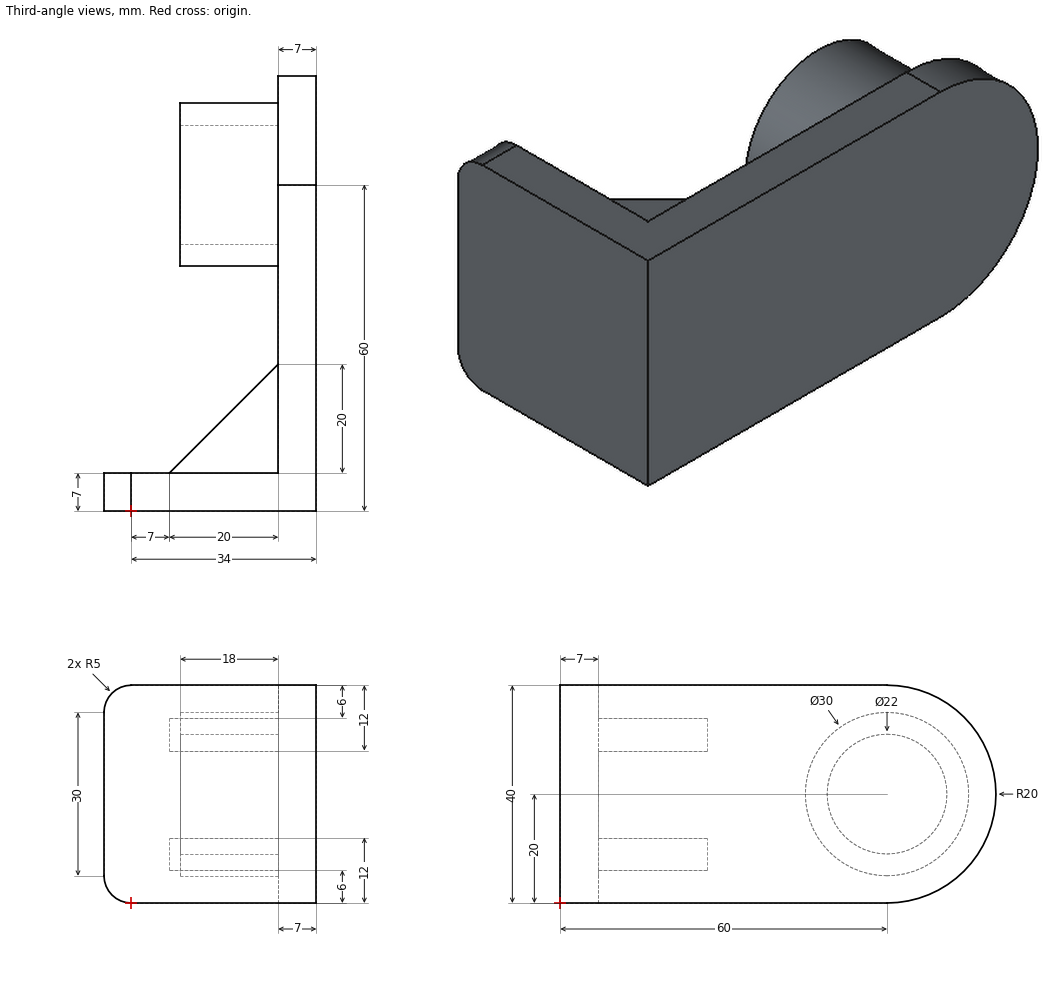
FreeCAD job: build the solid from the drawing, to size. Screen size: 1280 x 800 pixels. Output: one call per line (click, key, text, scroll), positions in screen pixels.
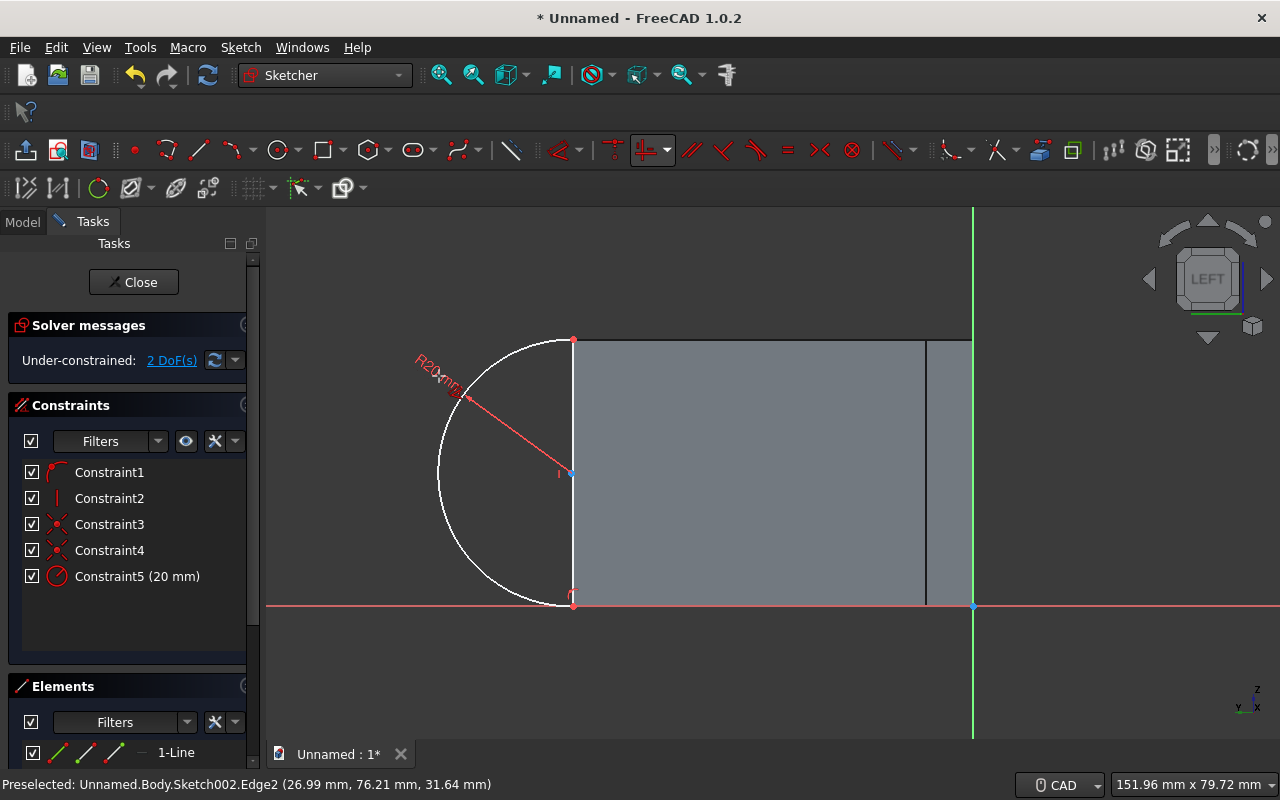
click(573, 606)
click(773, 640)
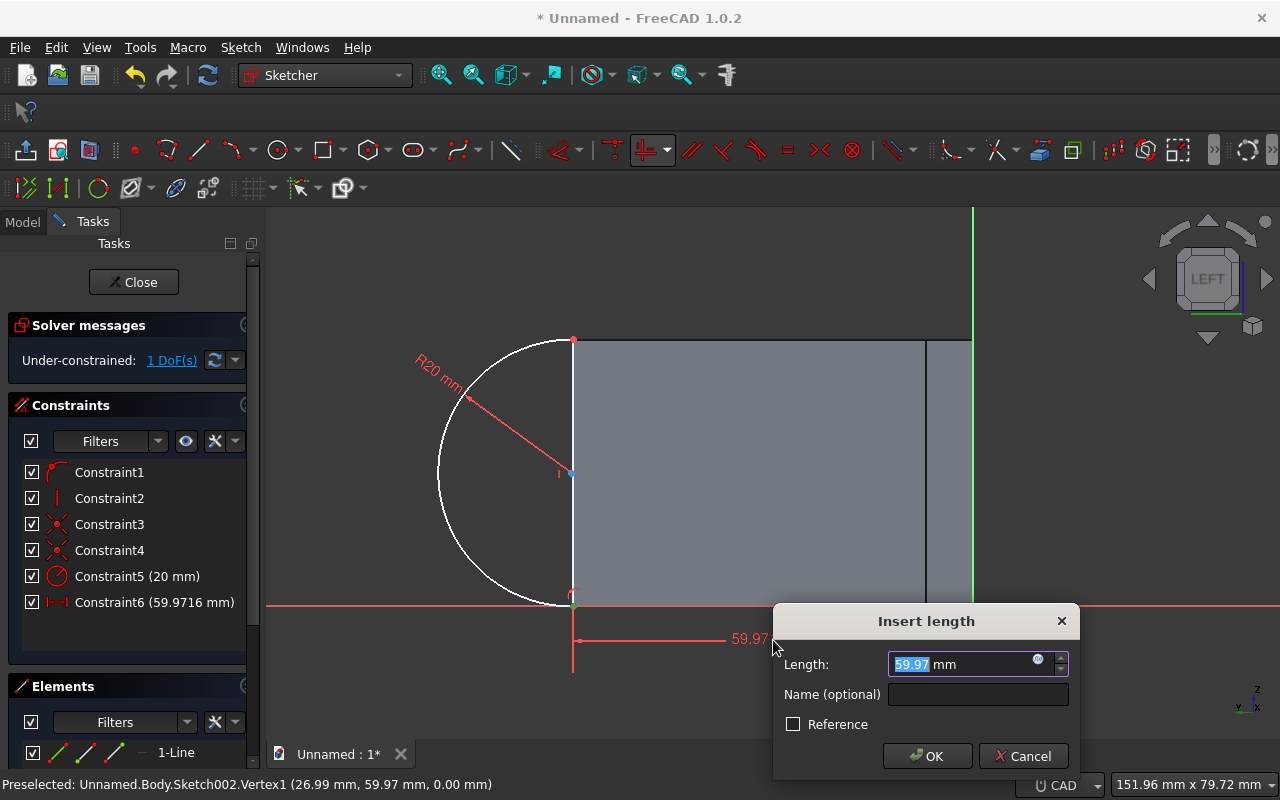
text(60)
key(Return)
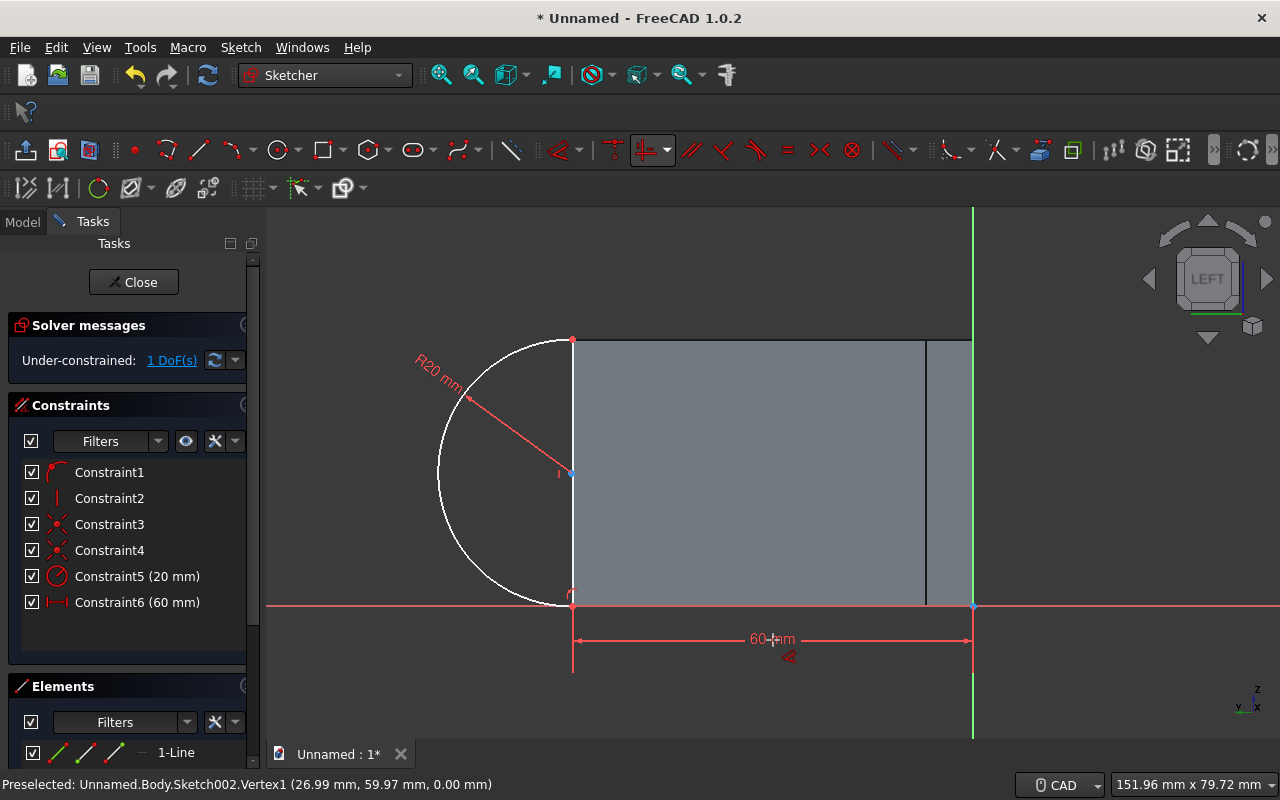
click(572, 473)
click(680, 640)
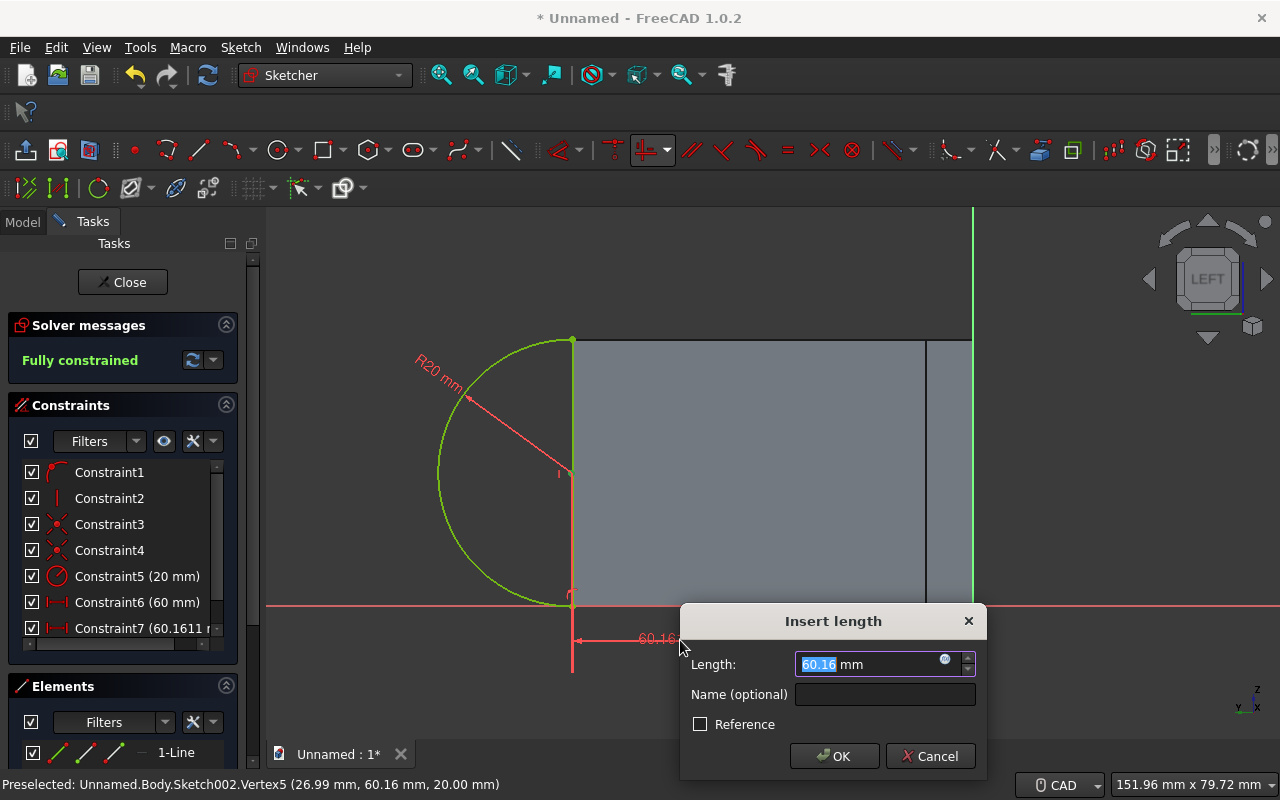
text(60)
key(Return)
key(Escape)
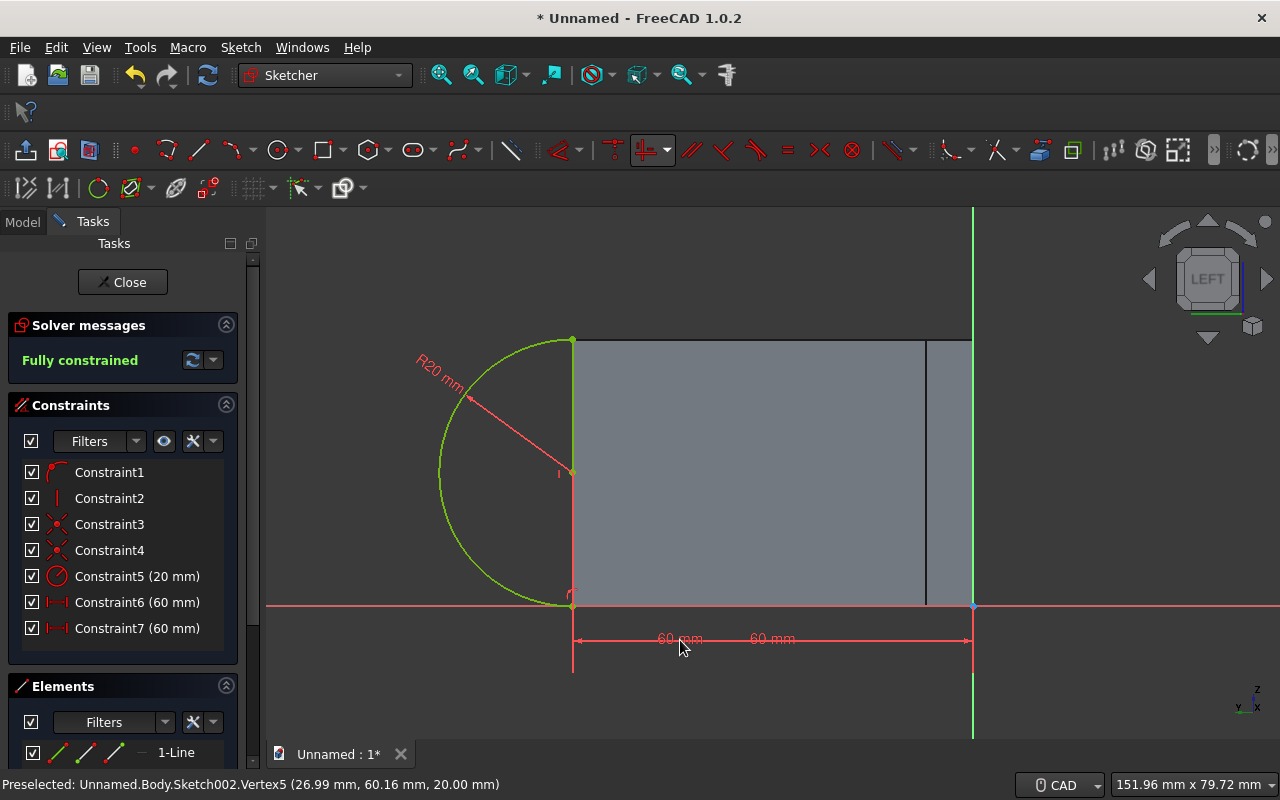
click(123, 282)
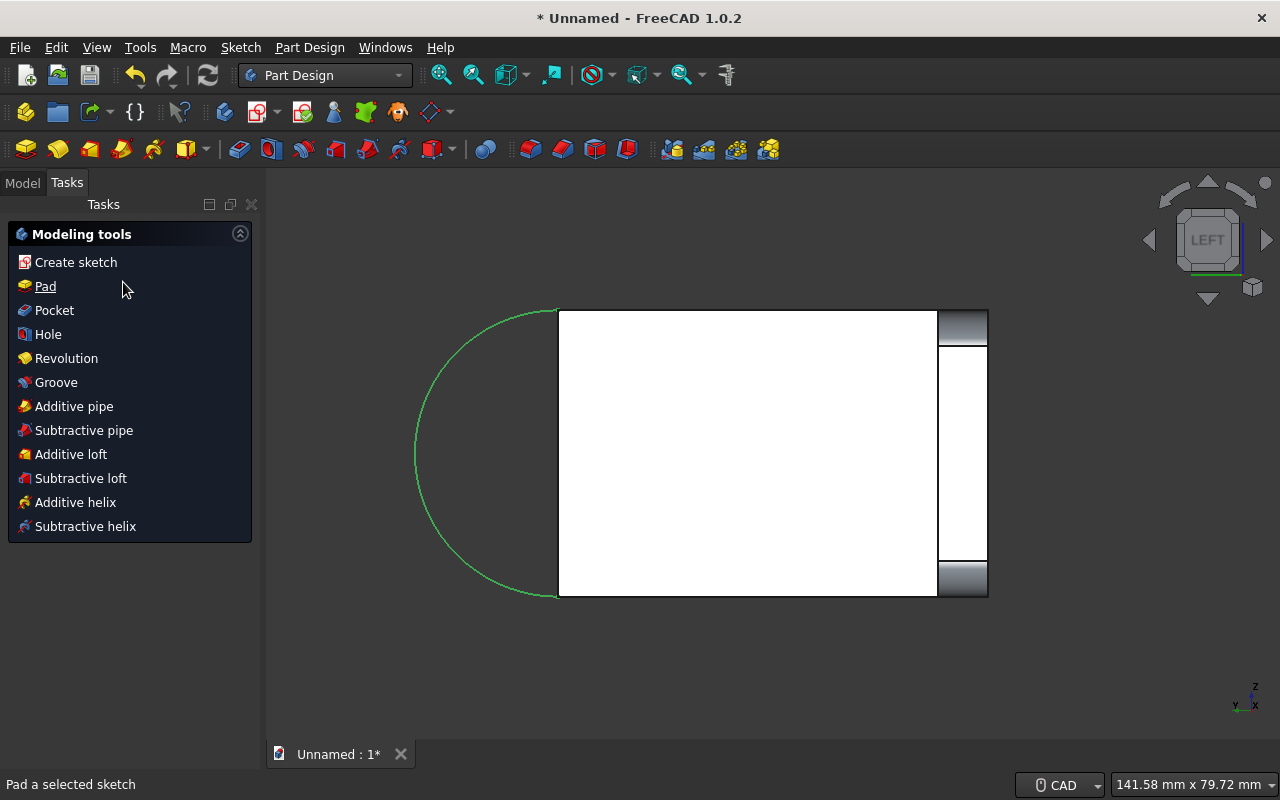
click(26, 150)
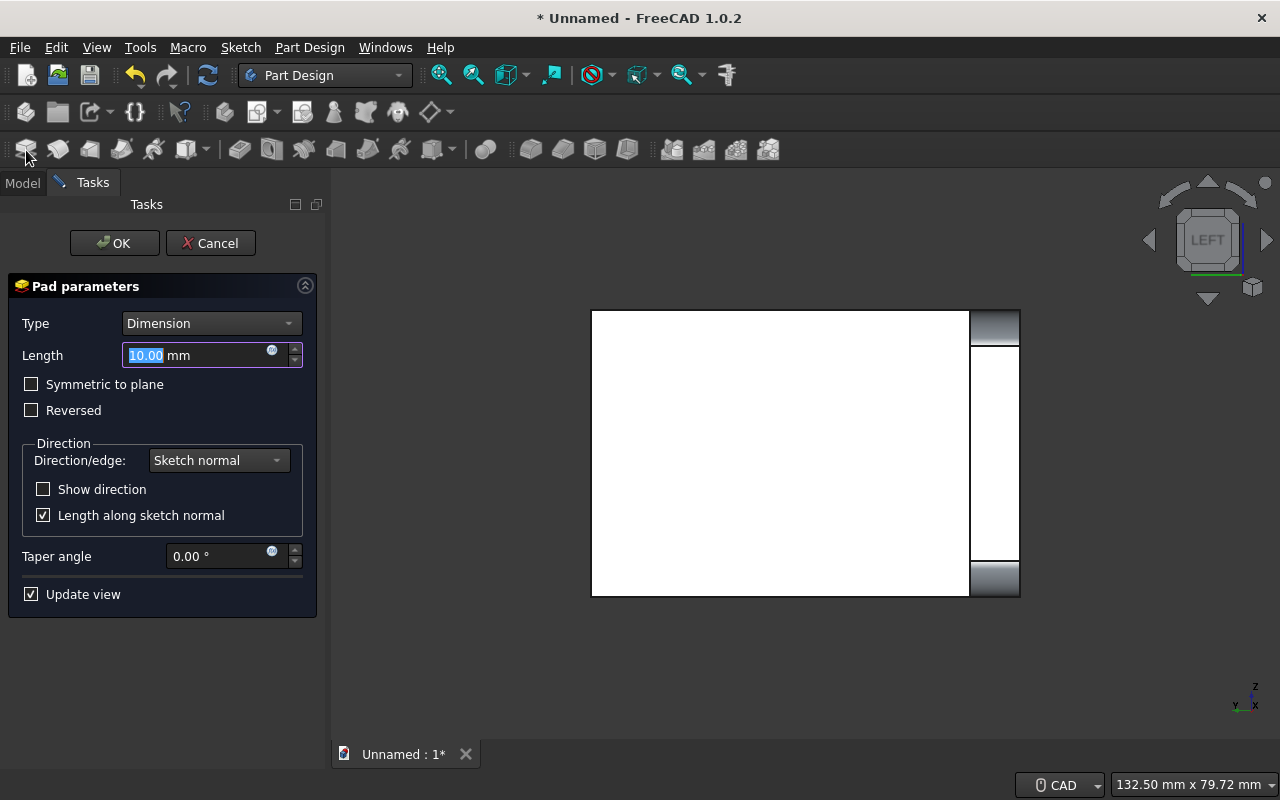
text(7)
key(Tab)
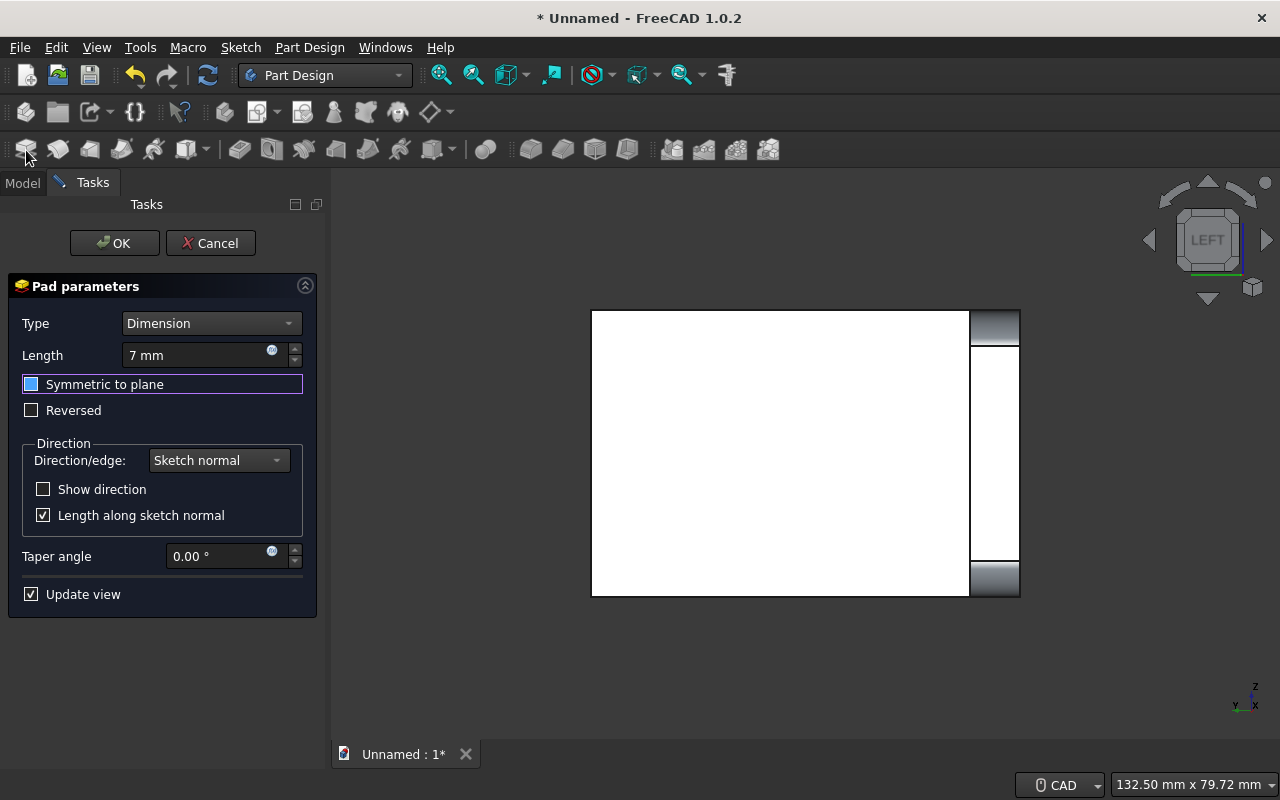
click(30, 410)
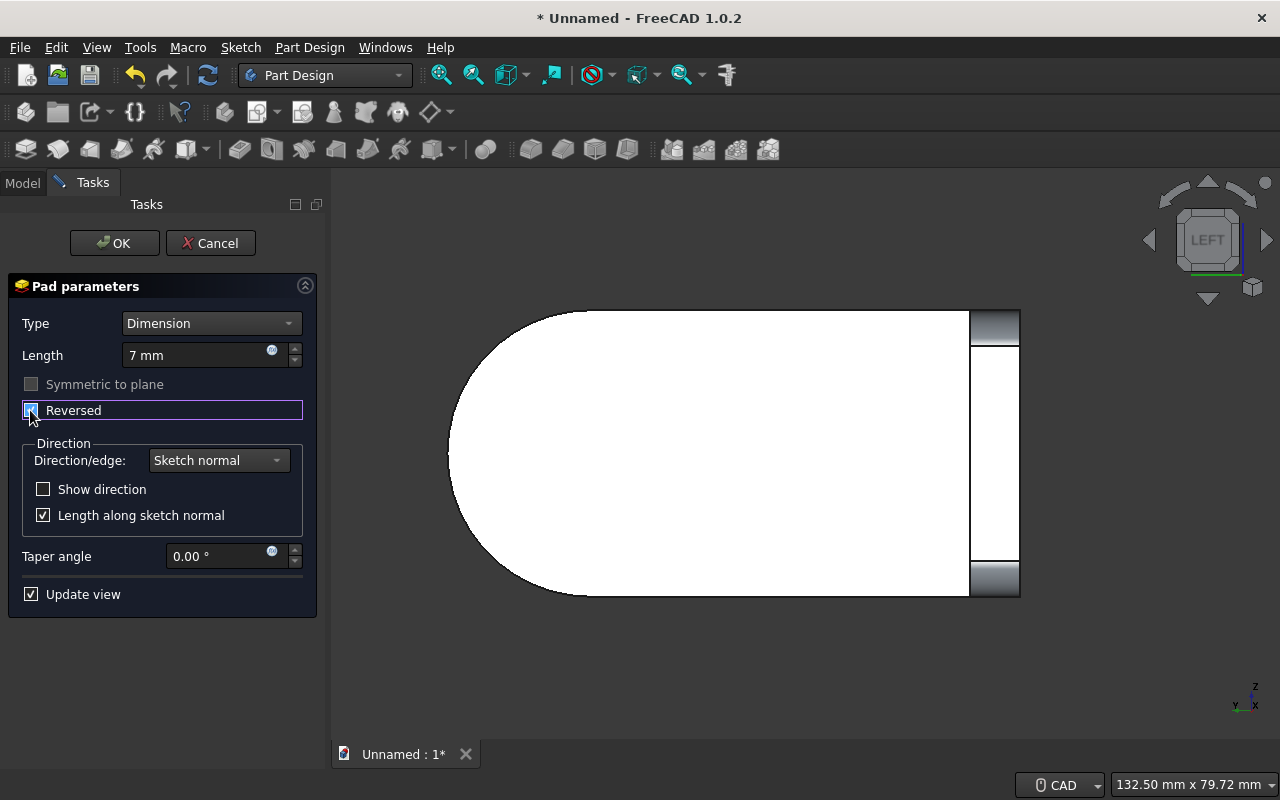
click(115, 243)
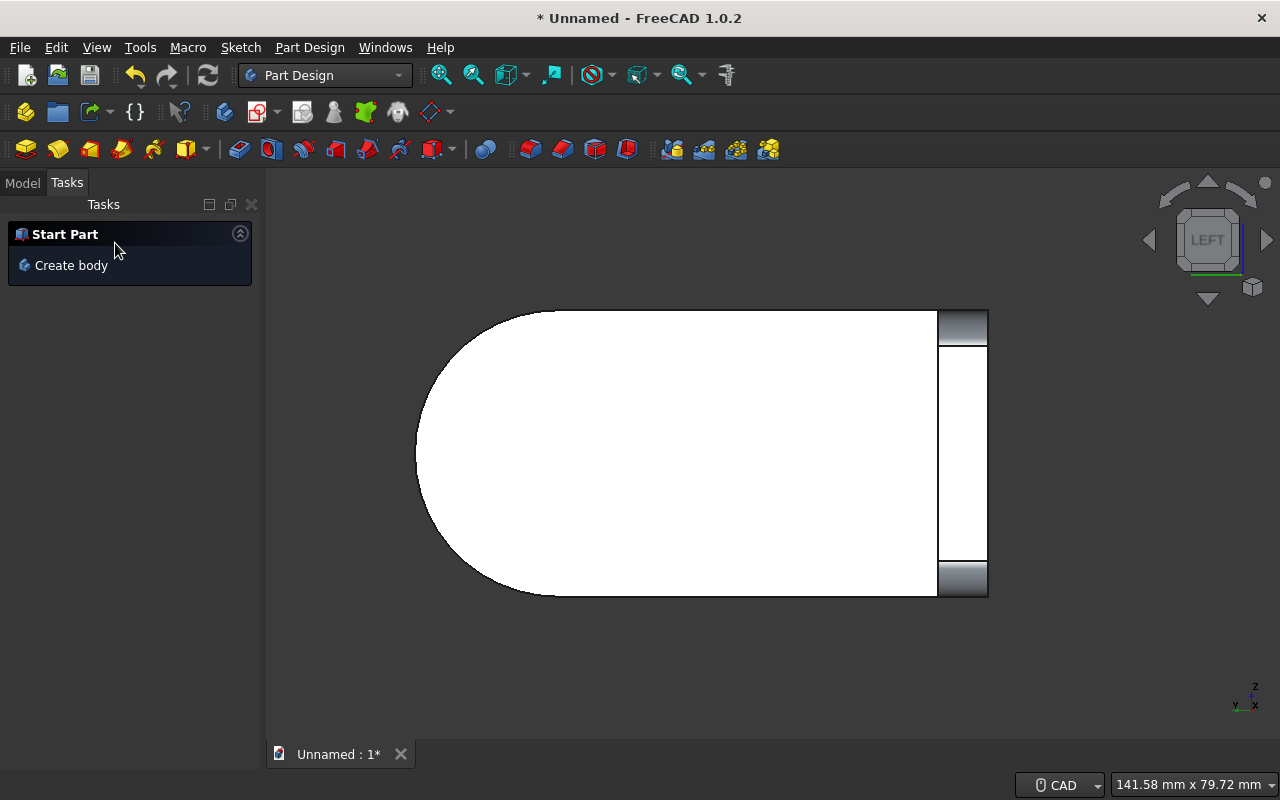
click(602, 453)